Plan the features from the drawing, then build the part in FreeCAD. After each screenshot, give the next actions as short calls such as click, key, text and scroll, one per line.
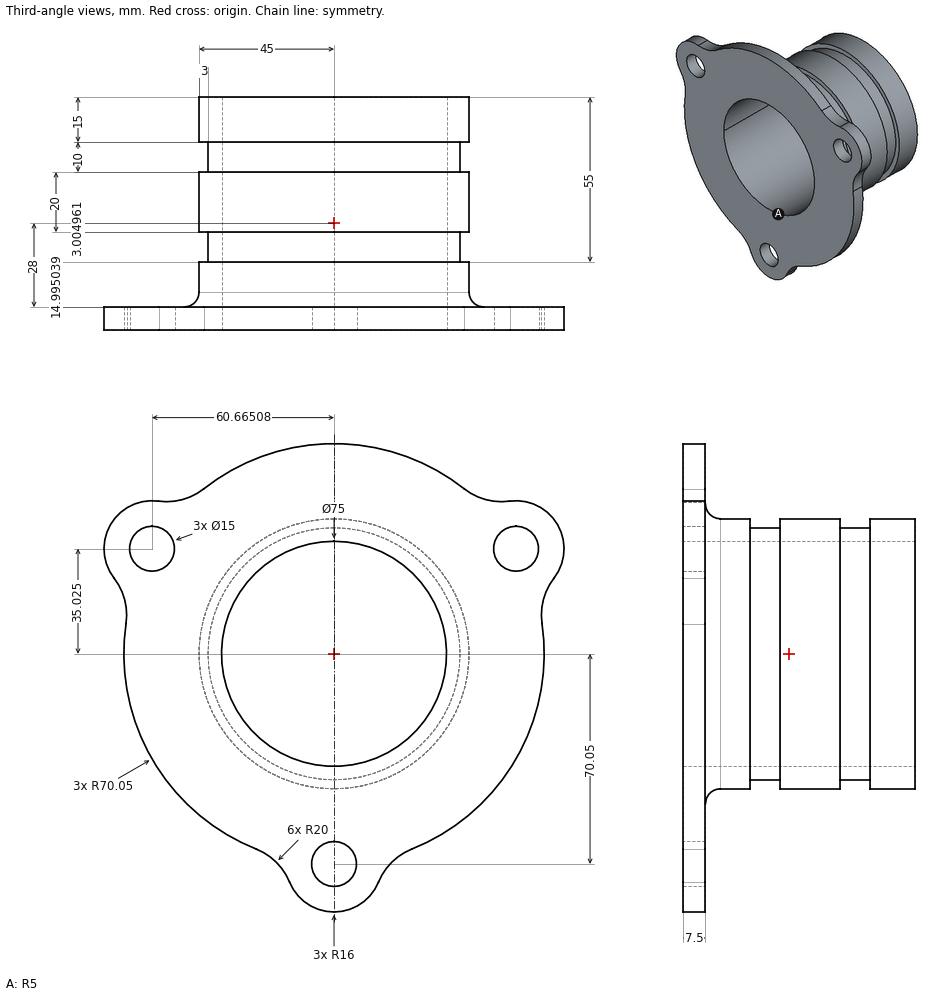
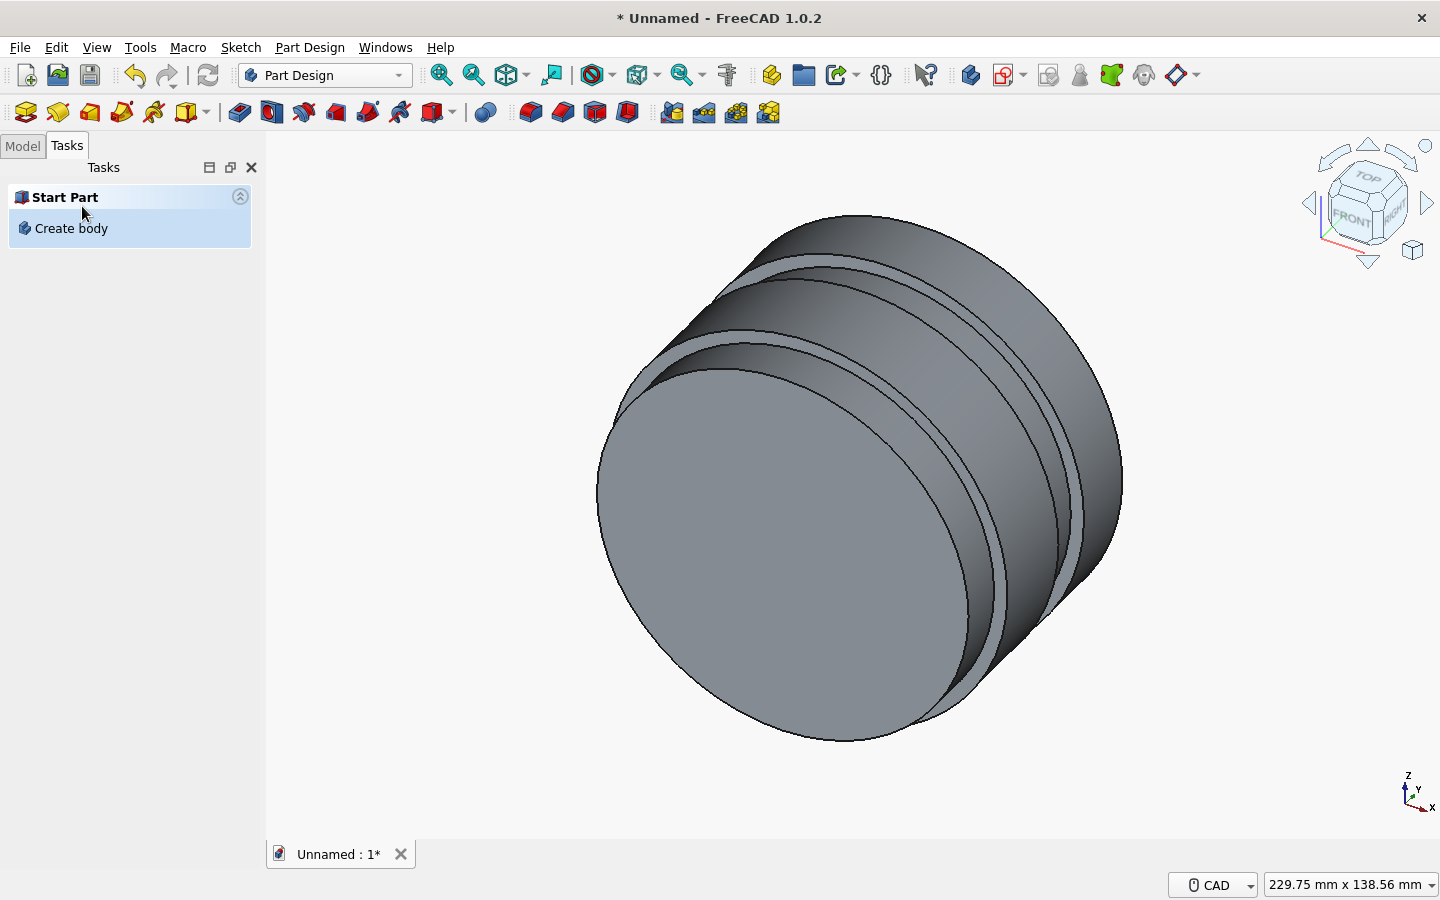
key(4)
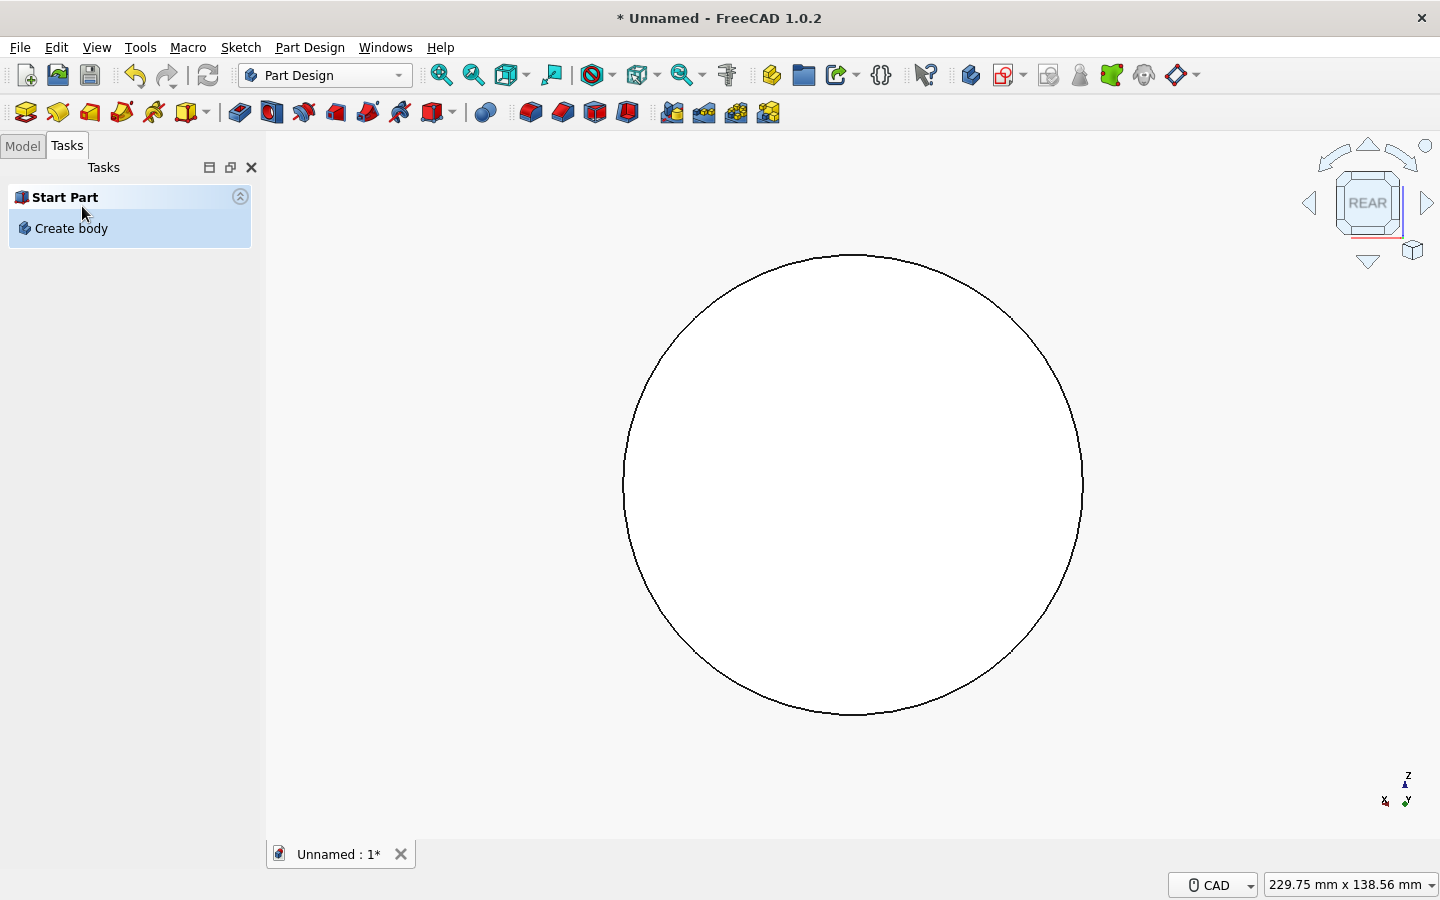
click(853, 484)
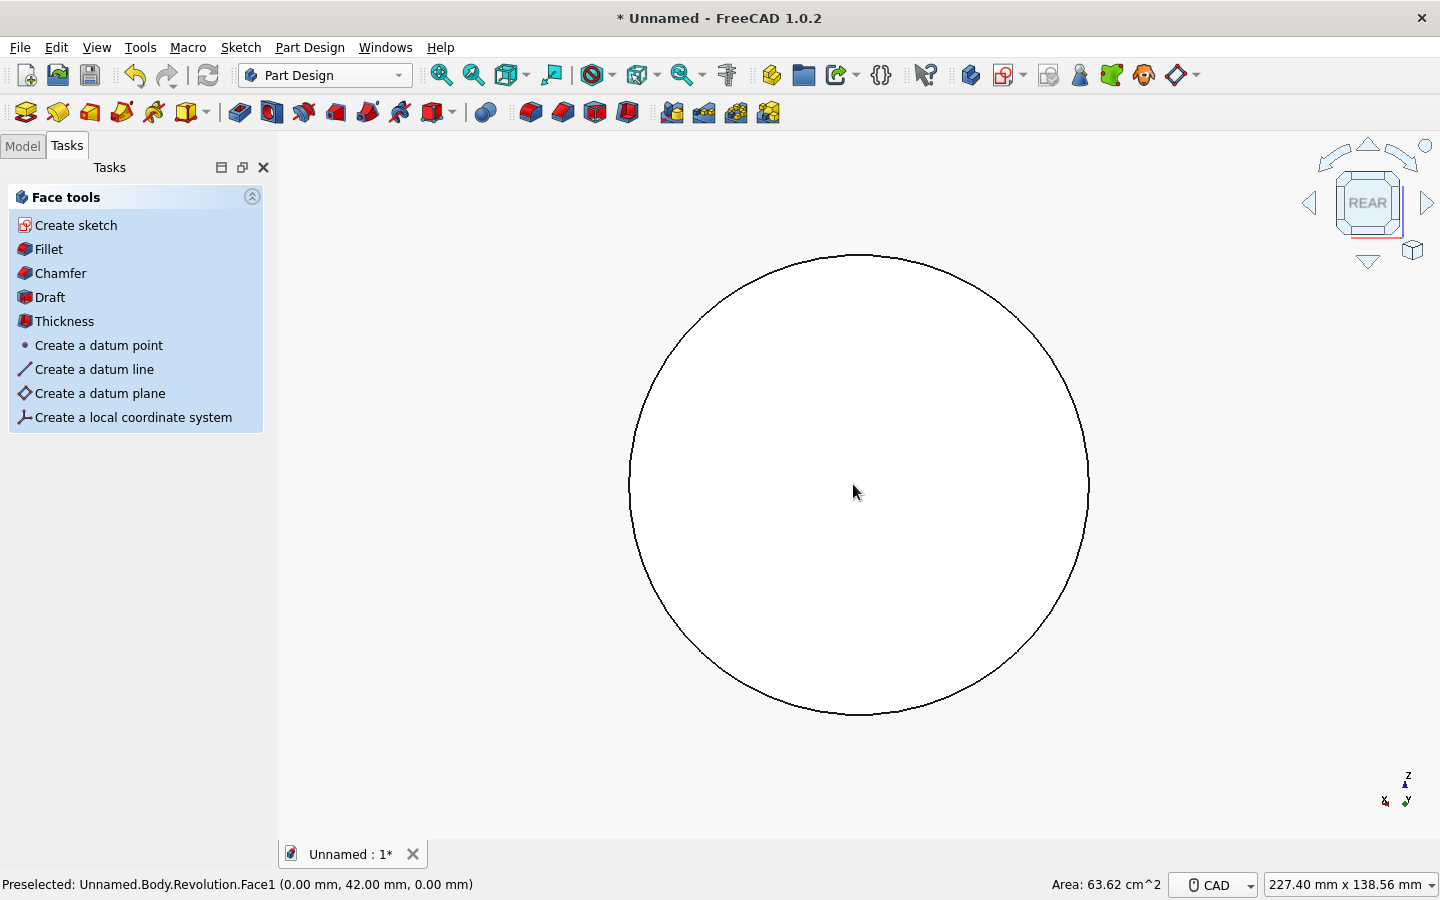
click(1004, 76)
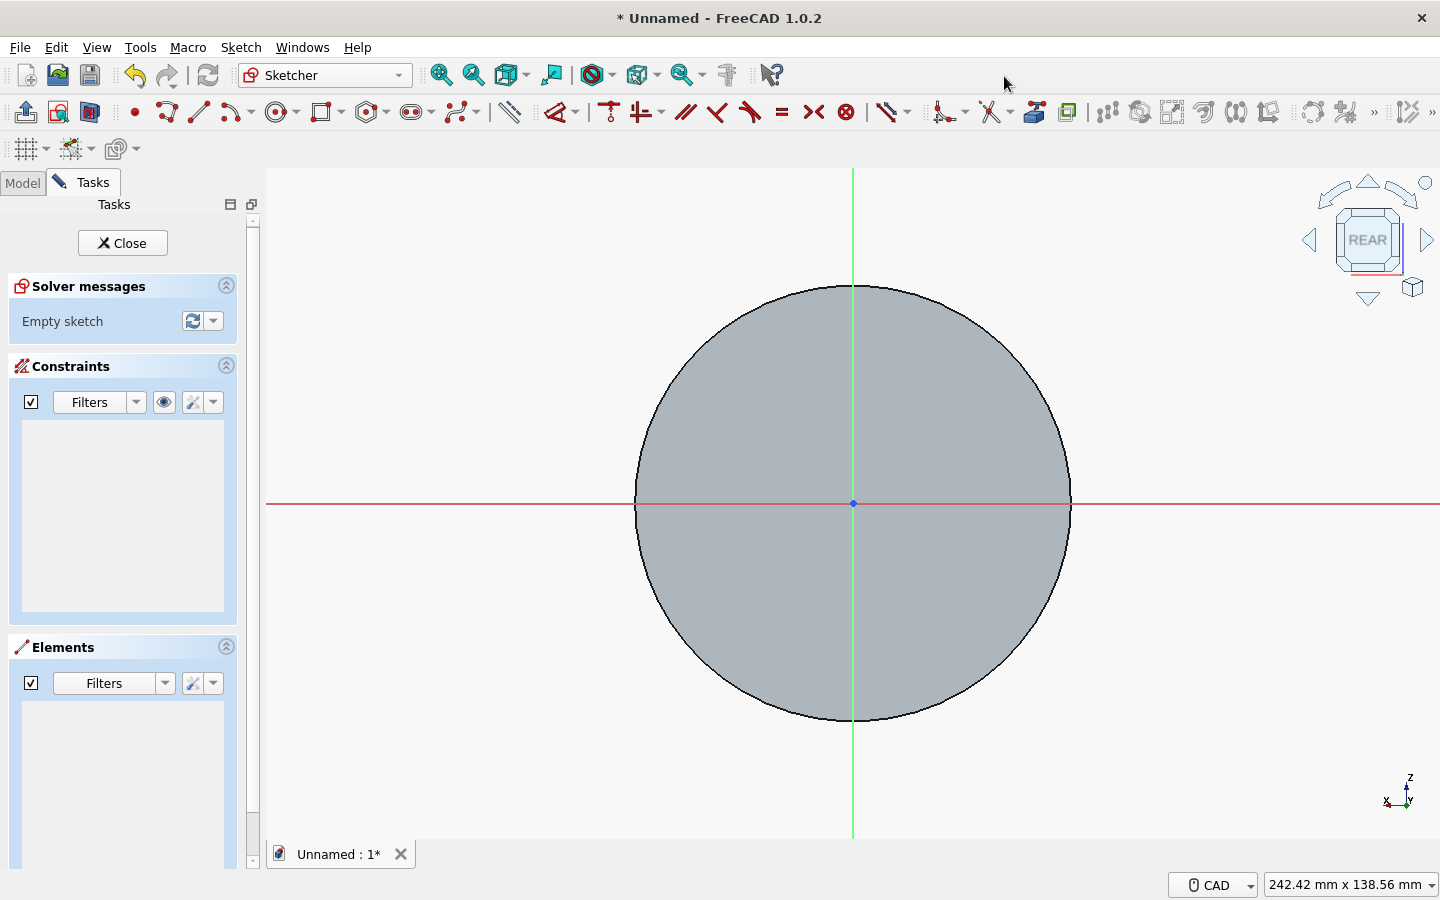
key(g)
key(c)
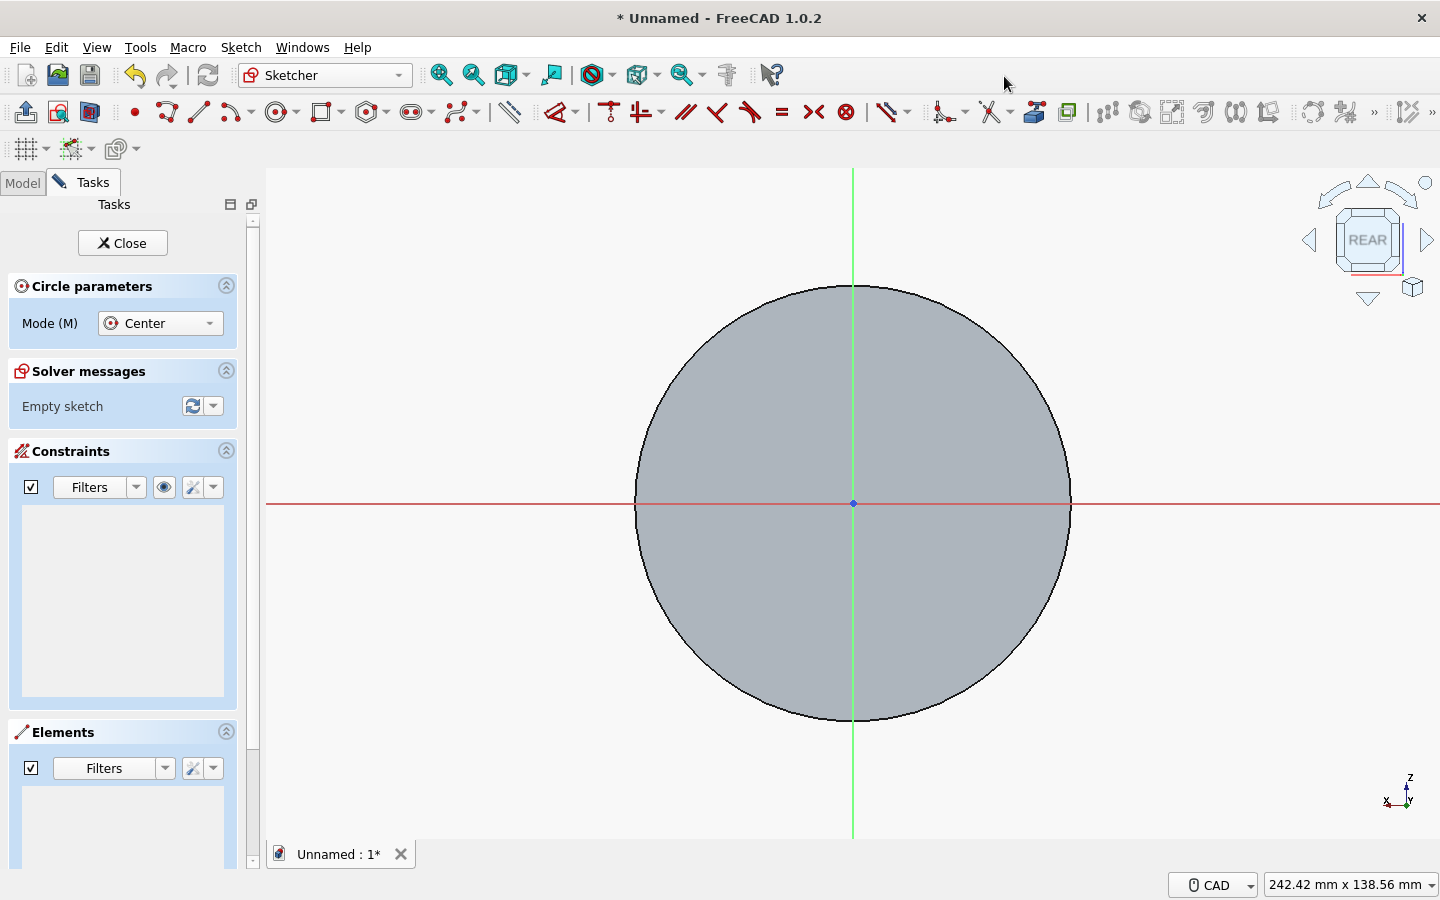
click(853, 503)
click(981, 375)
key(Escape)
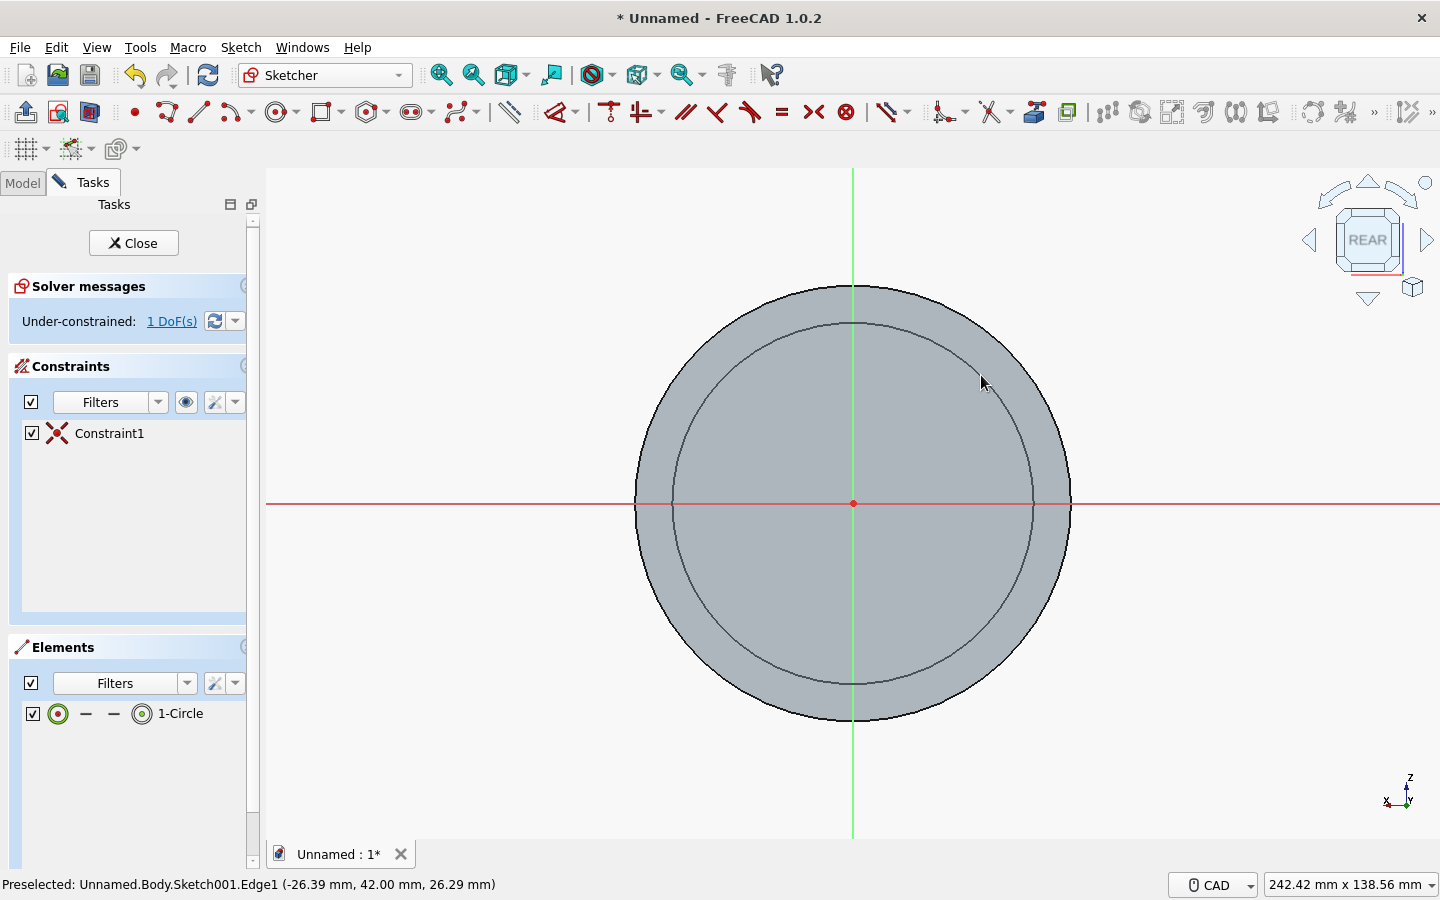
key(d)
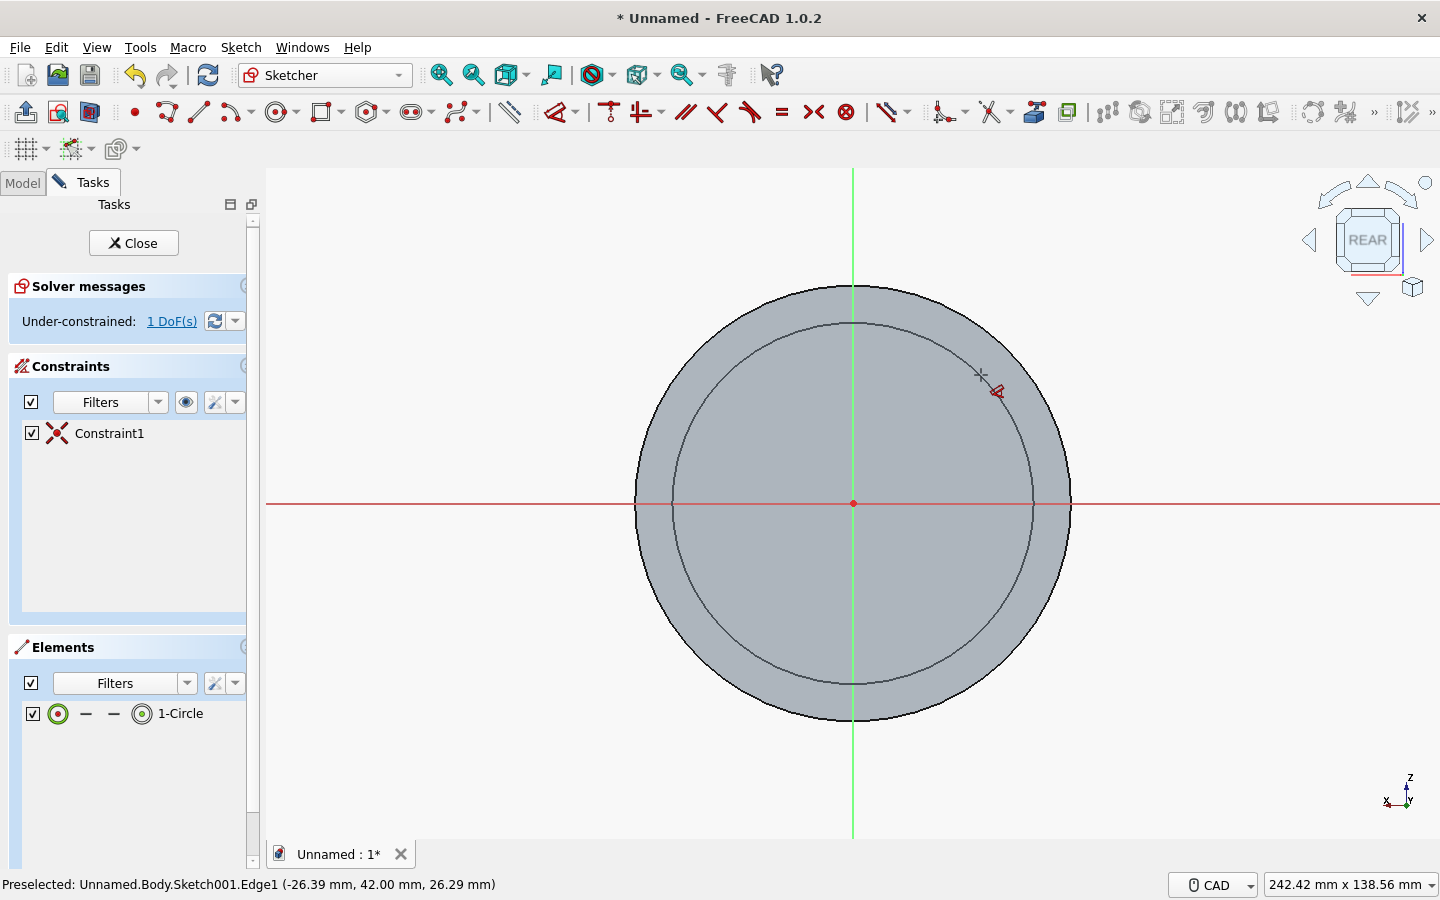
click(980, 375)
click(1002, 352)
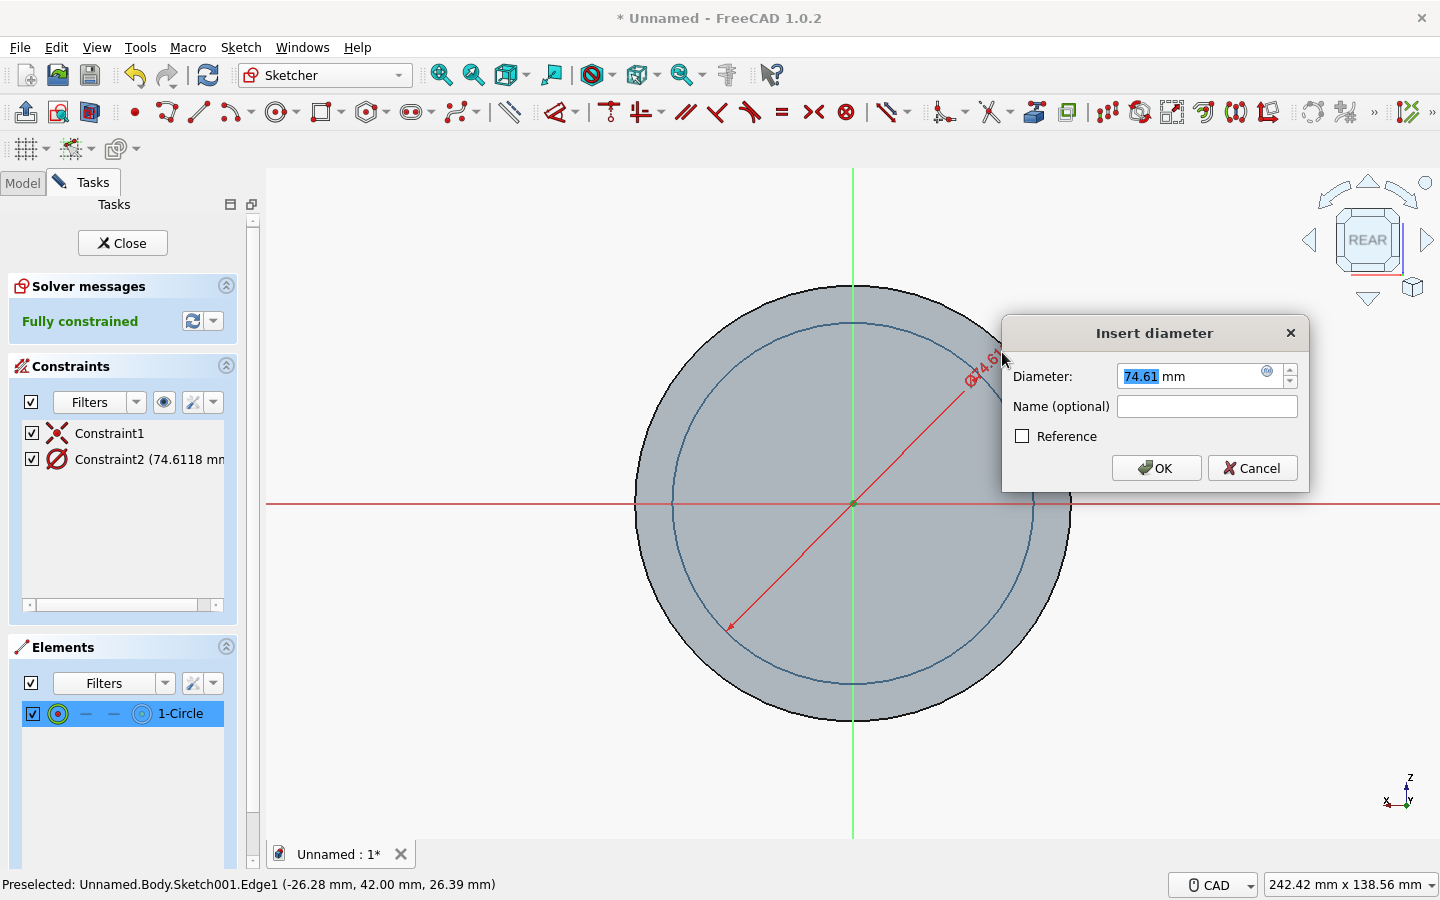
text(75)
key(Return)
key(Escape)